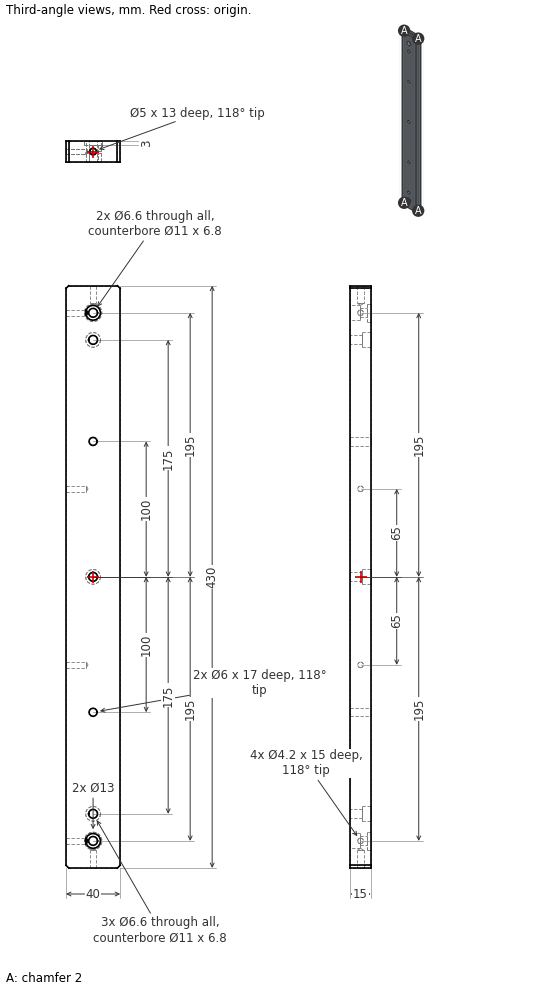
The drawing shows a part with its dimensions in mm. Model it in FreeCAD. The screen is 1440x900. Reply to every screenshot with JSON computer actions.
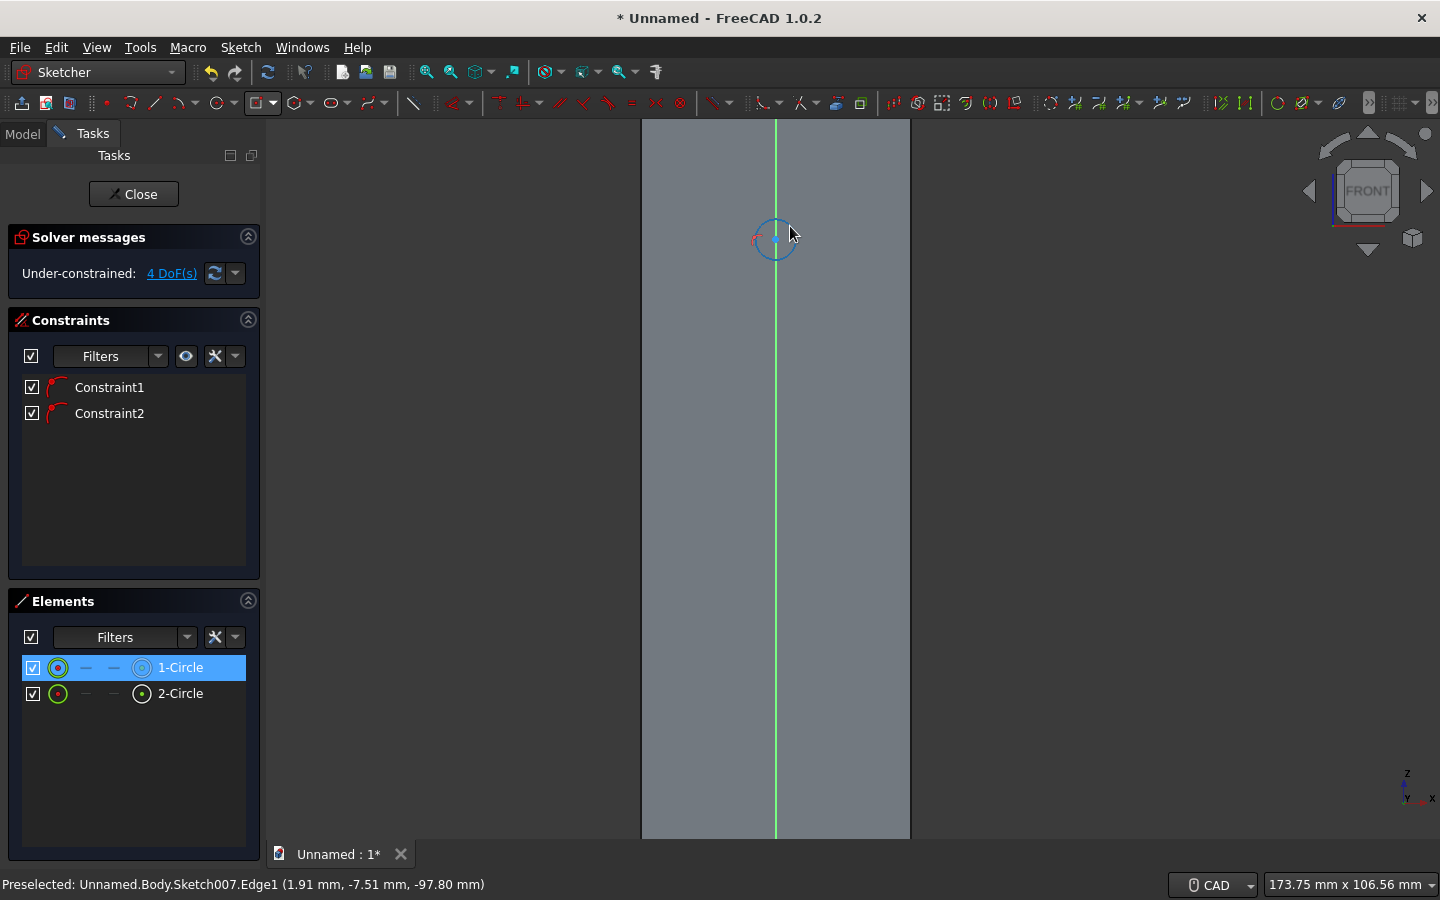
{"action": "left_click", "coordinate": [790, 225]}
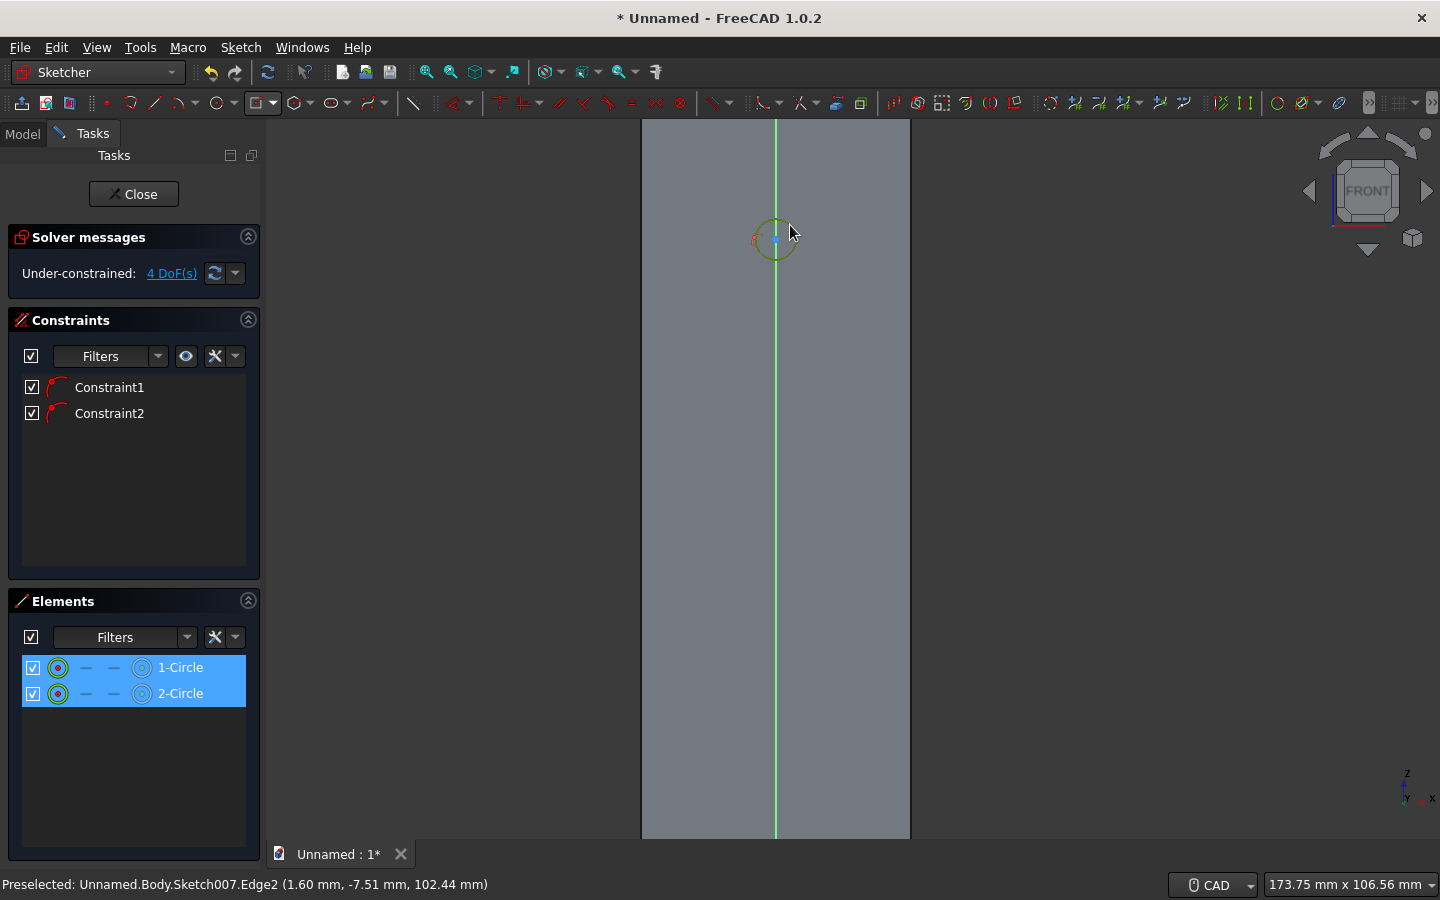
{"action": "left_click", "coordinate": [632, 104]}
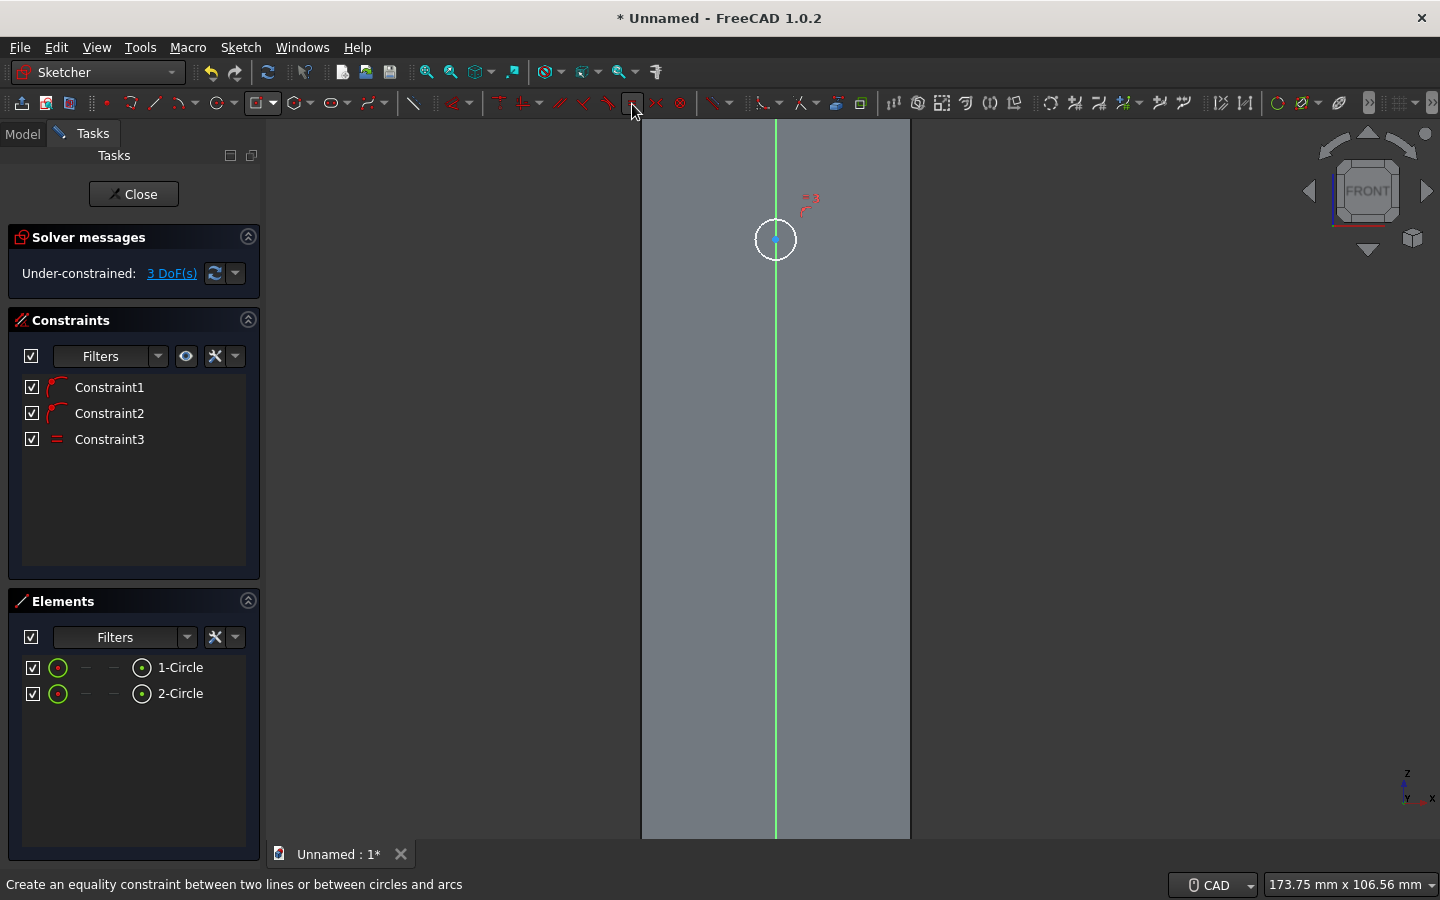
{"action": "left_click", "coordinate": [452, 104]}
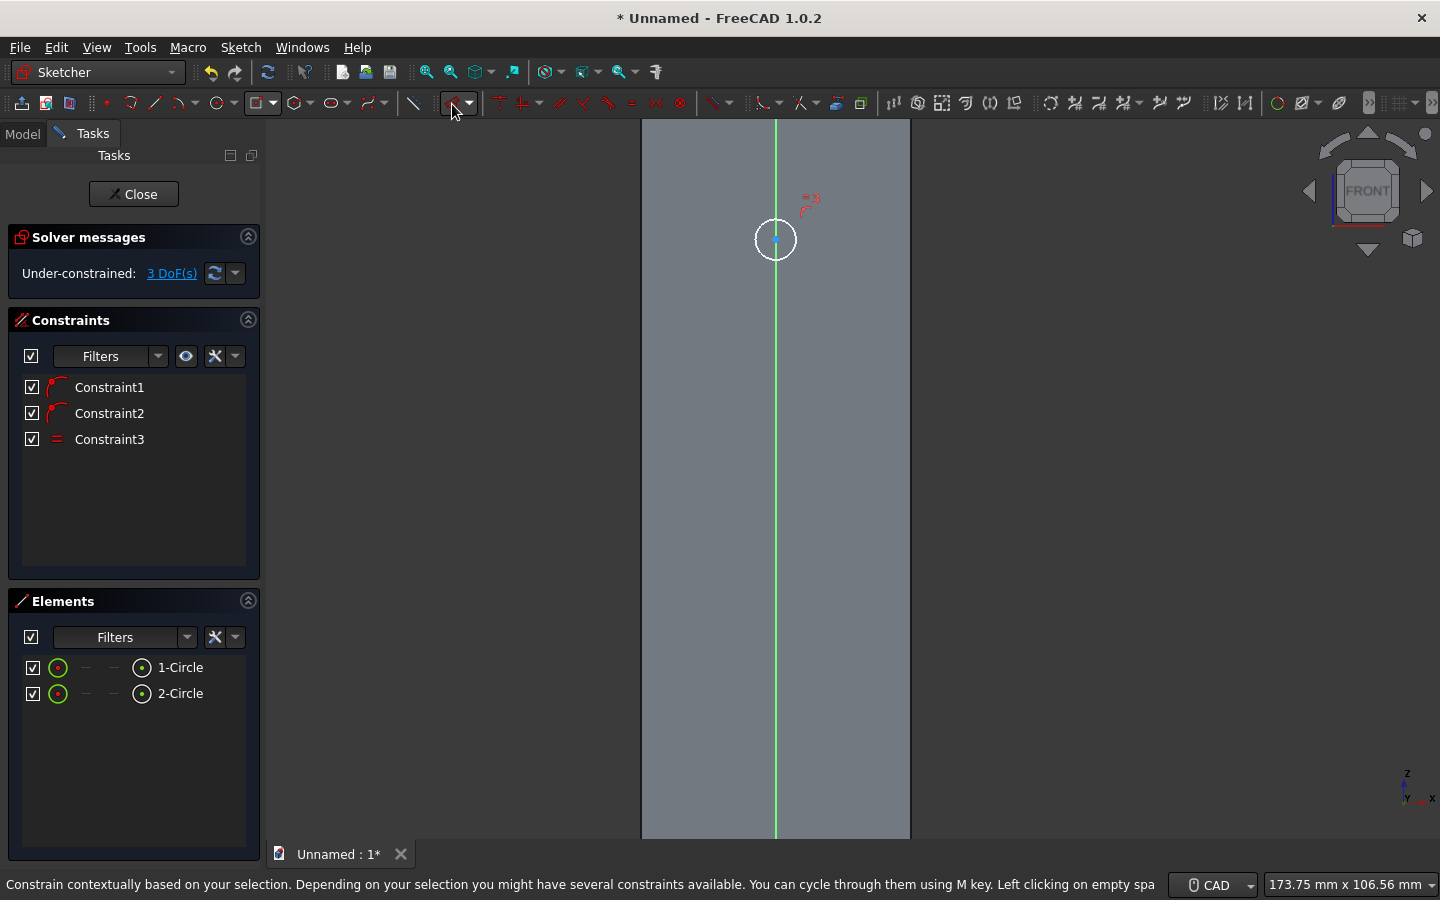
{"action": "scroll", "coordinate": [790, 225], "scroll_direction": "down", "scroll_amount": 5}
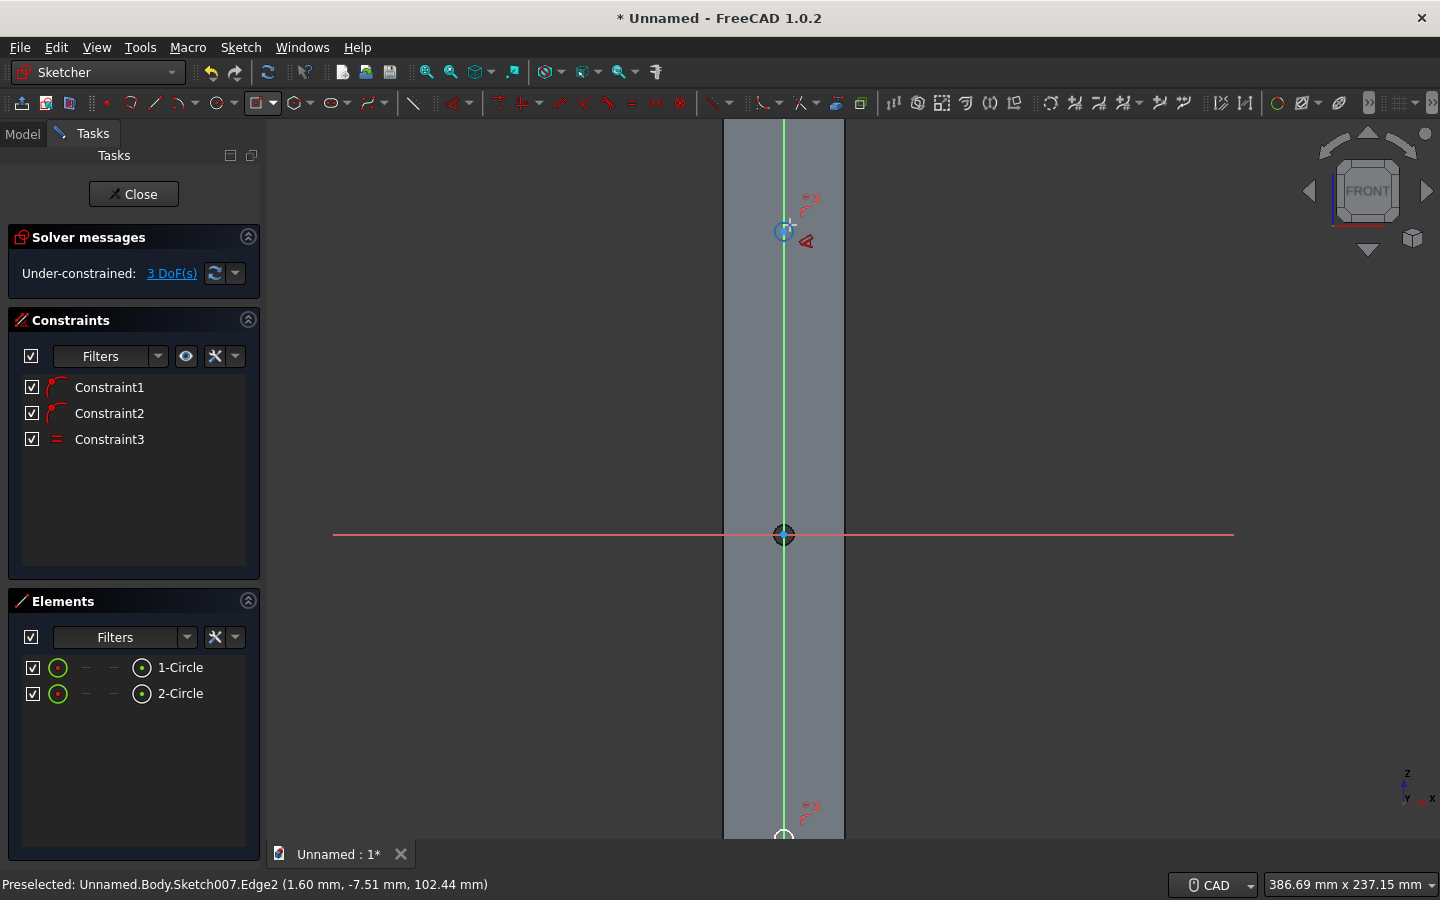
{"action": "scroll", "coordinate": [790, 722], "scroll_direction": "up", "scroll_amount": 5}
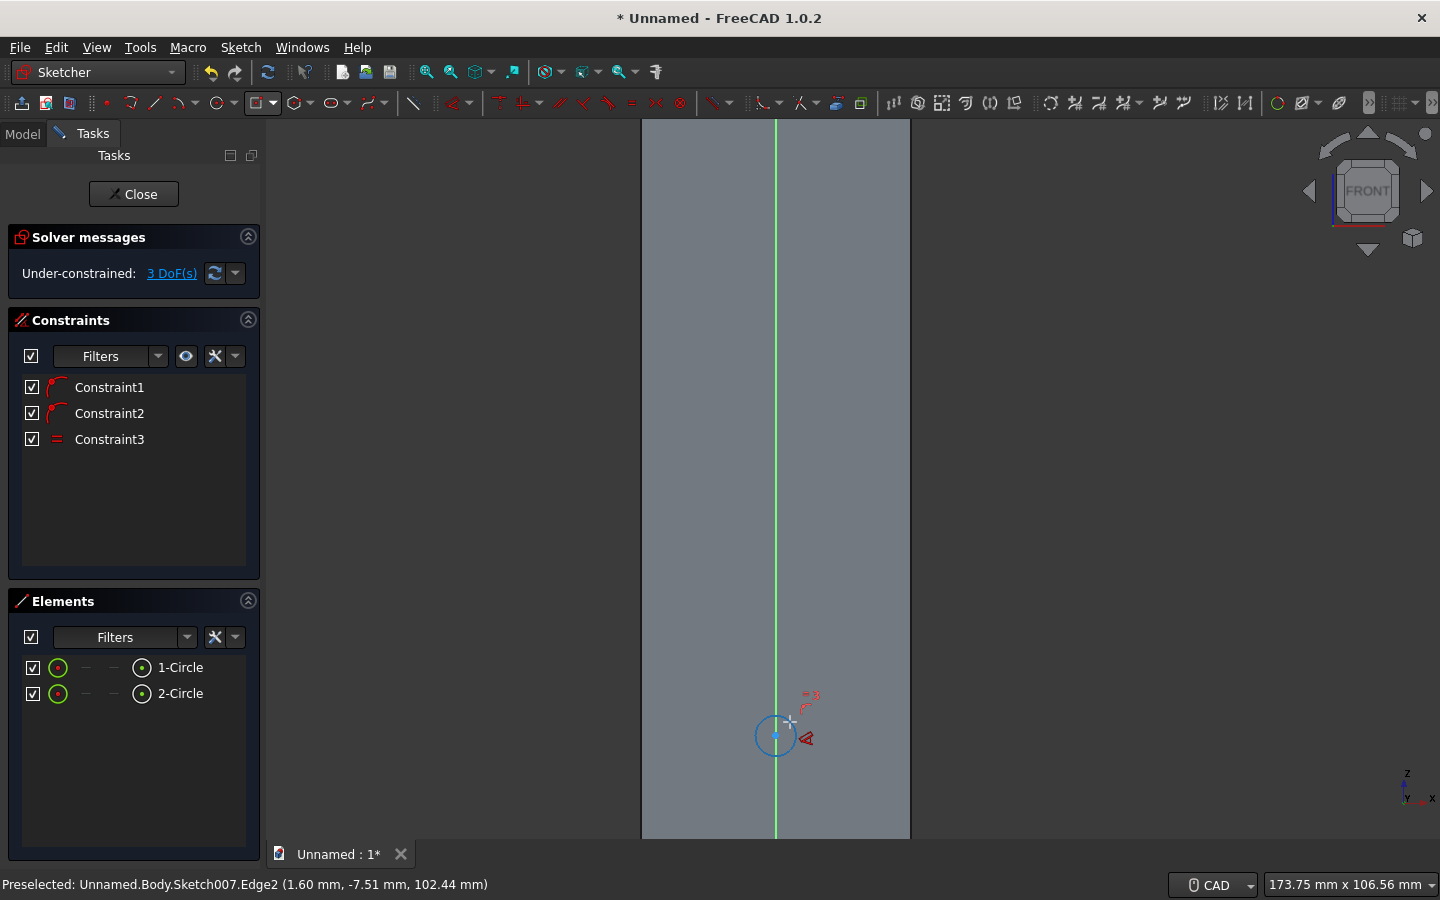
{"action": "left_click", "coordinate": [790, 722]}
{"action": "left_click", "coordinate": [813, 700]}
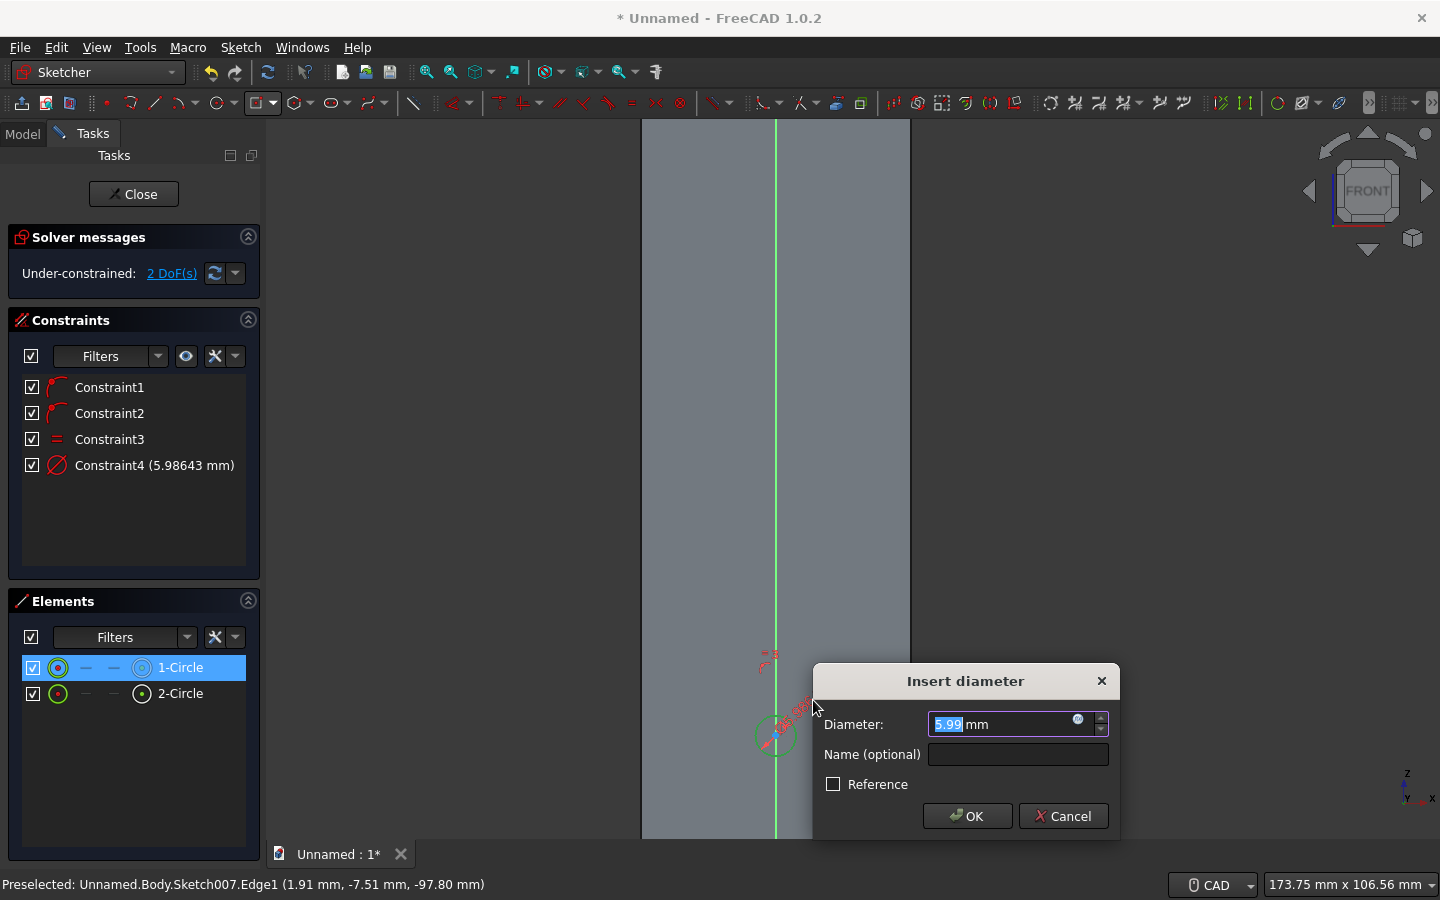
{"action": "type", "text": "6"}
{"action": "key", "text": "Return"}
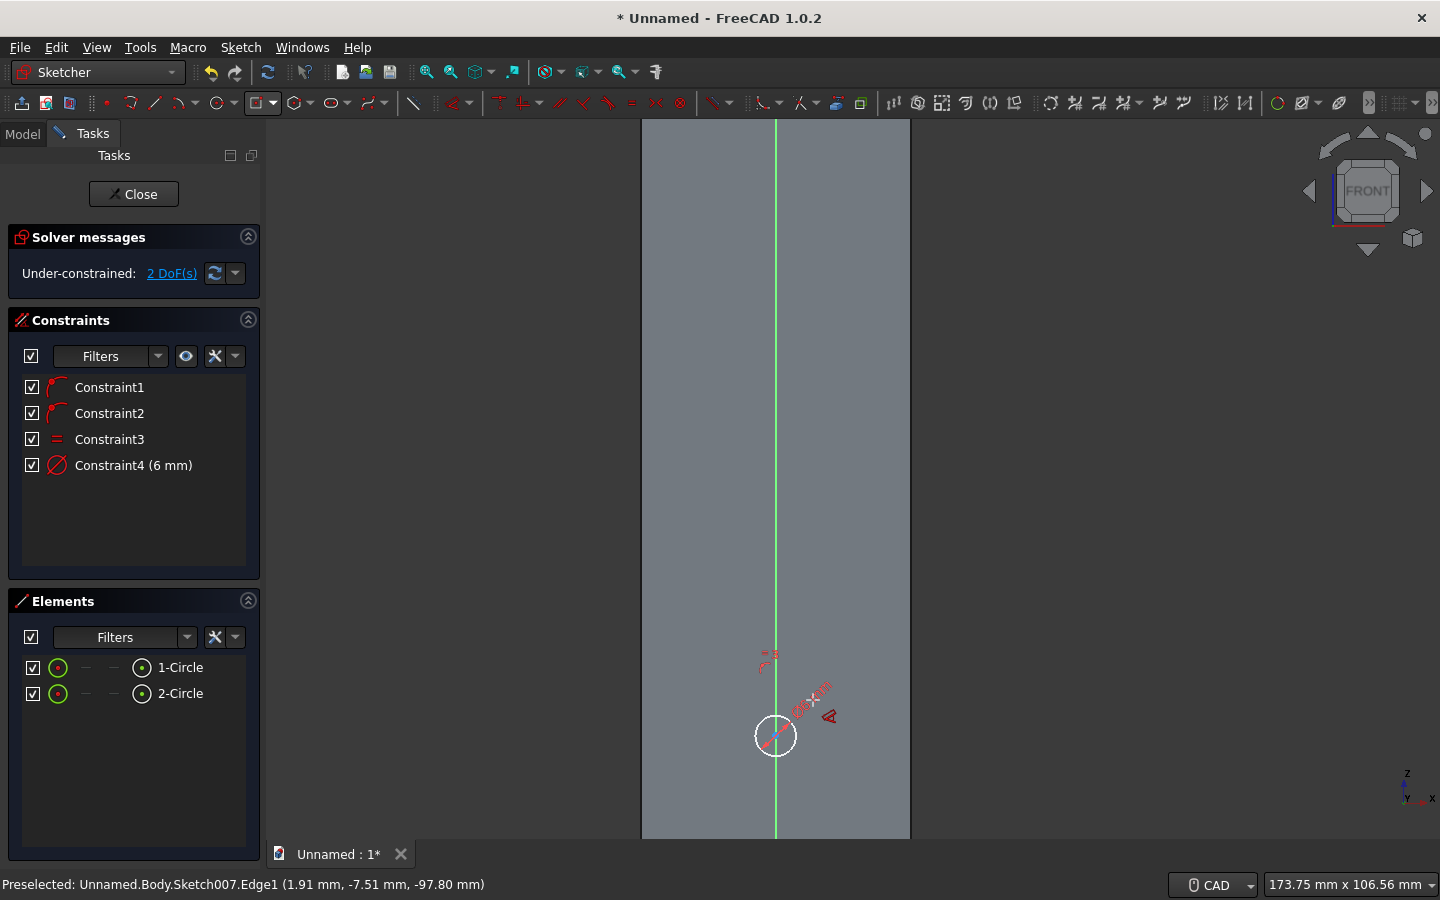
{"action": "left_click", "coordinate": [776, 736]}
{"action": "left_click", "coordinate": [810, 441]}